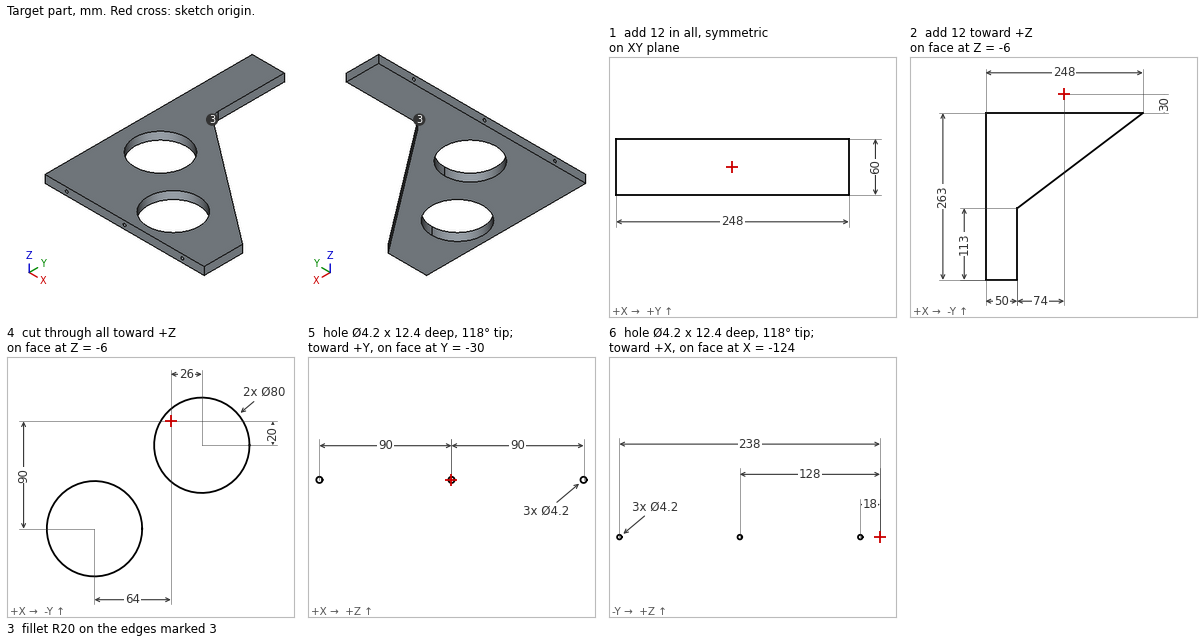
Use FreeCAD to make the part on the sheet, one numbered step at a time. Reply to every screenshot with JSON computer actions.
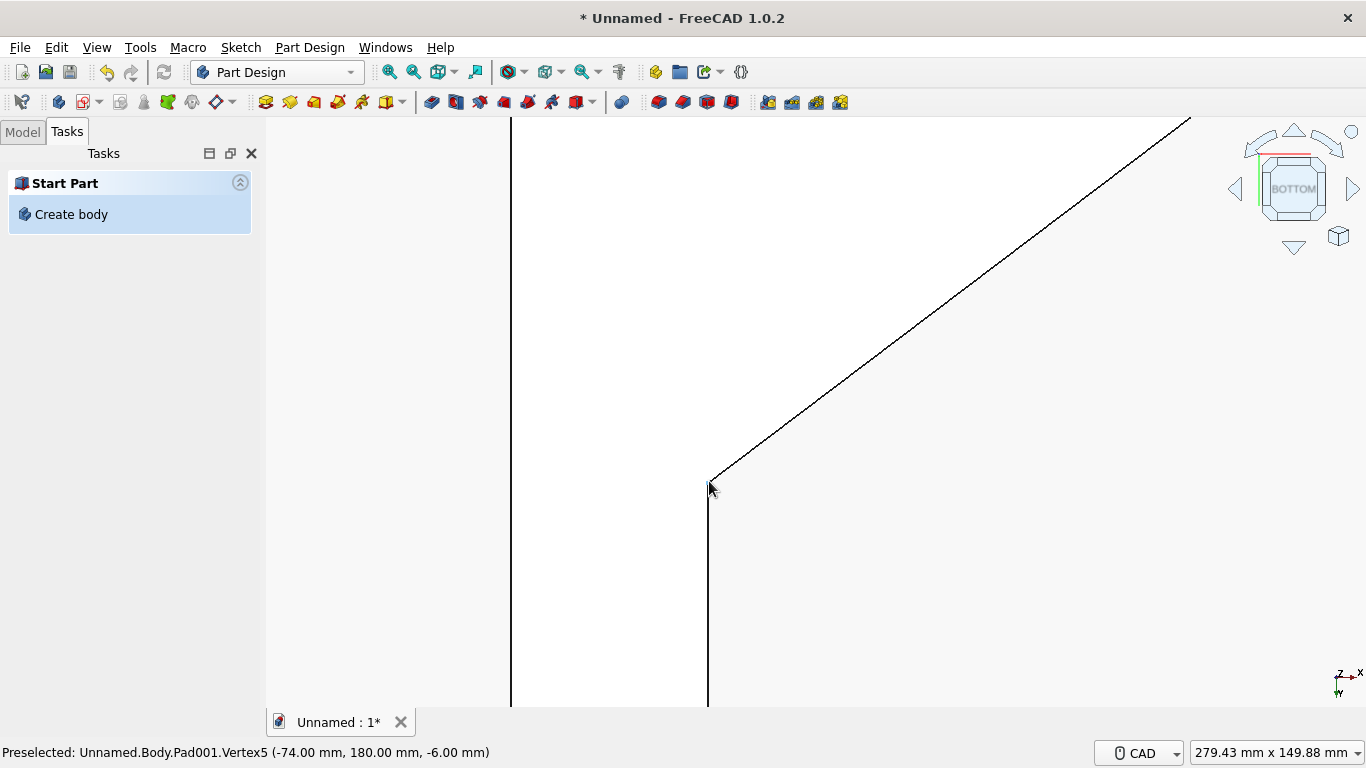
{"action": "key", "text": "v f"}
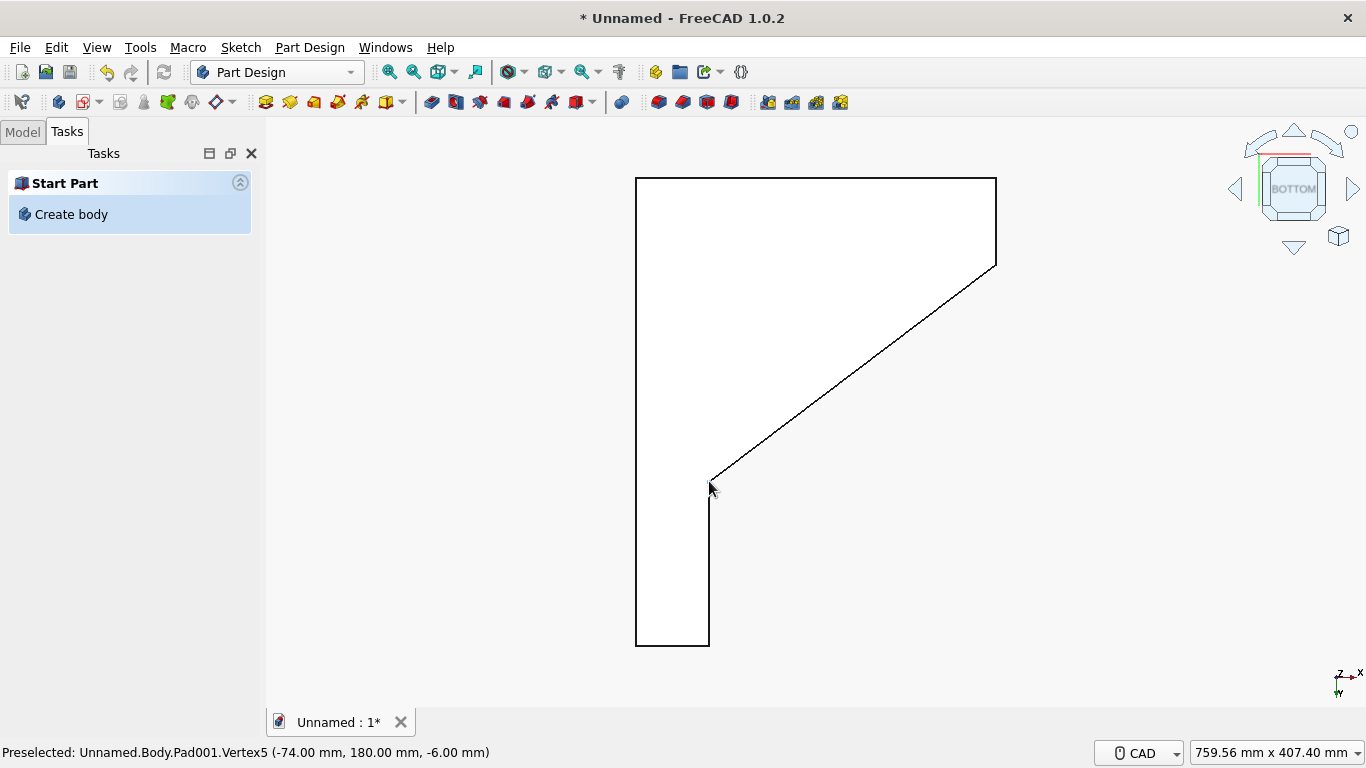
{"action": "key", "text": "0"}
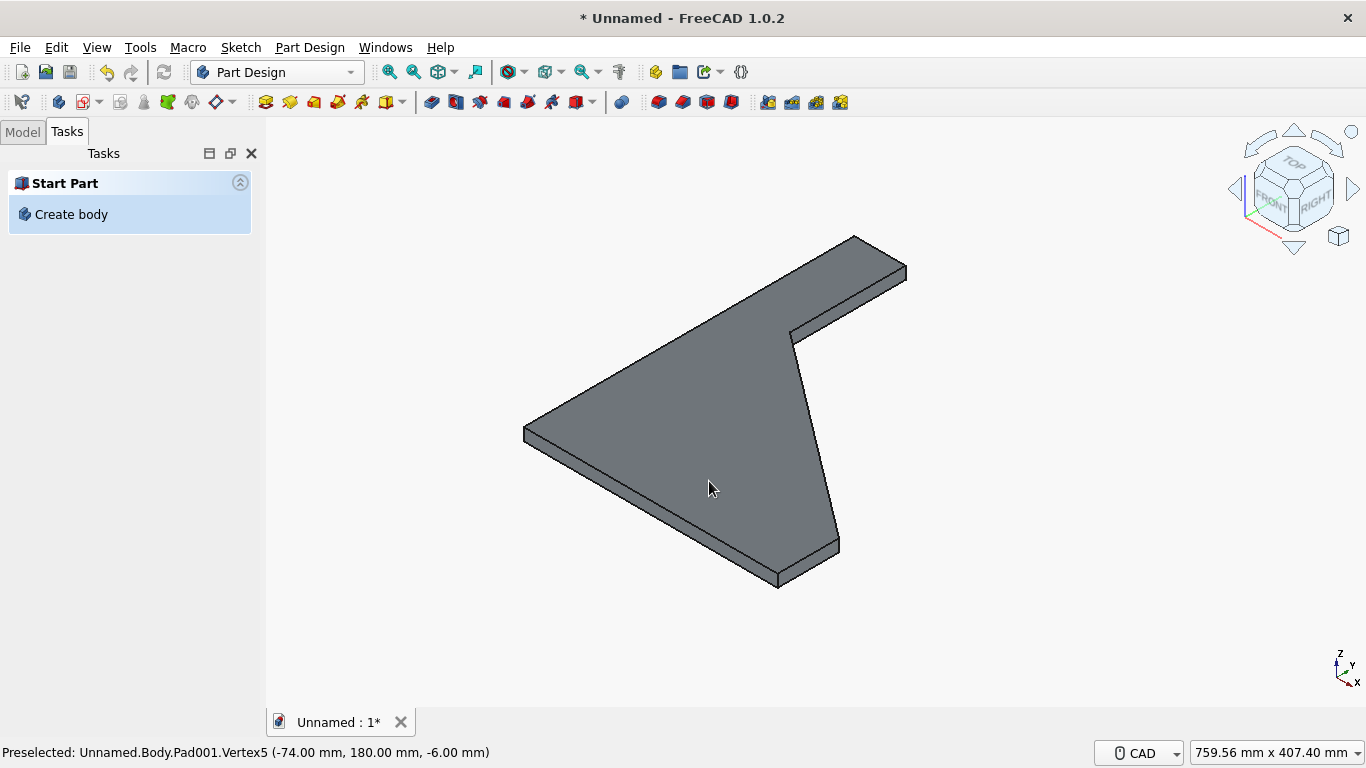
{"action": "scroll", "coordinate": [790, 339], "scroll_direction": "up", "scroll_amount": 5}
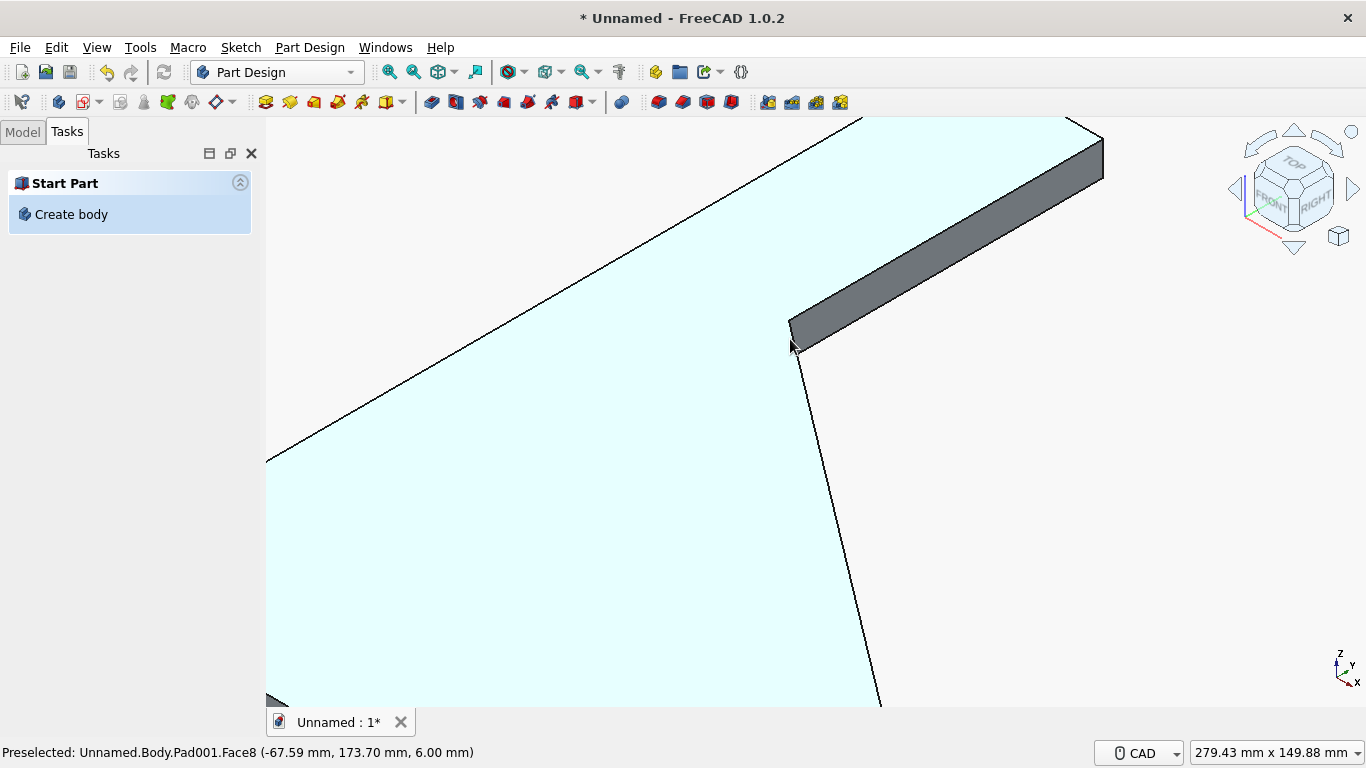
{"action": "key", "text": "v f"}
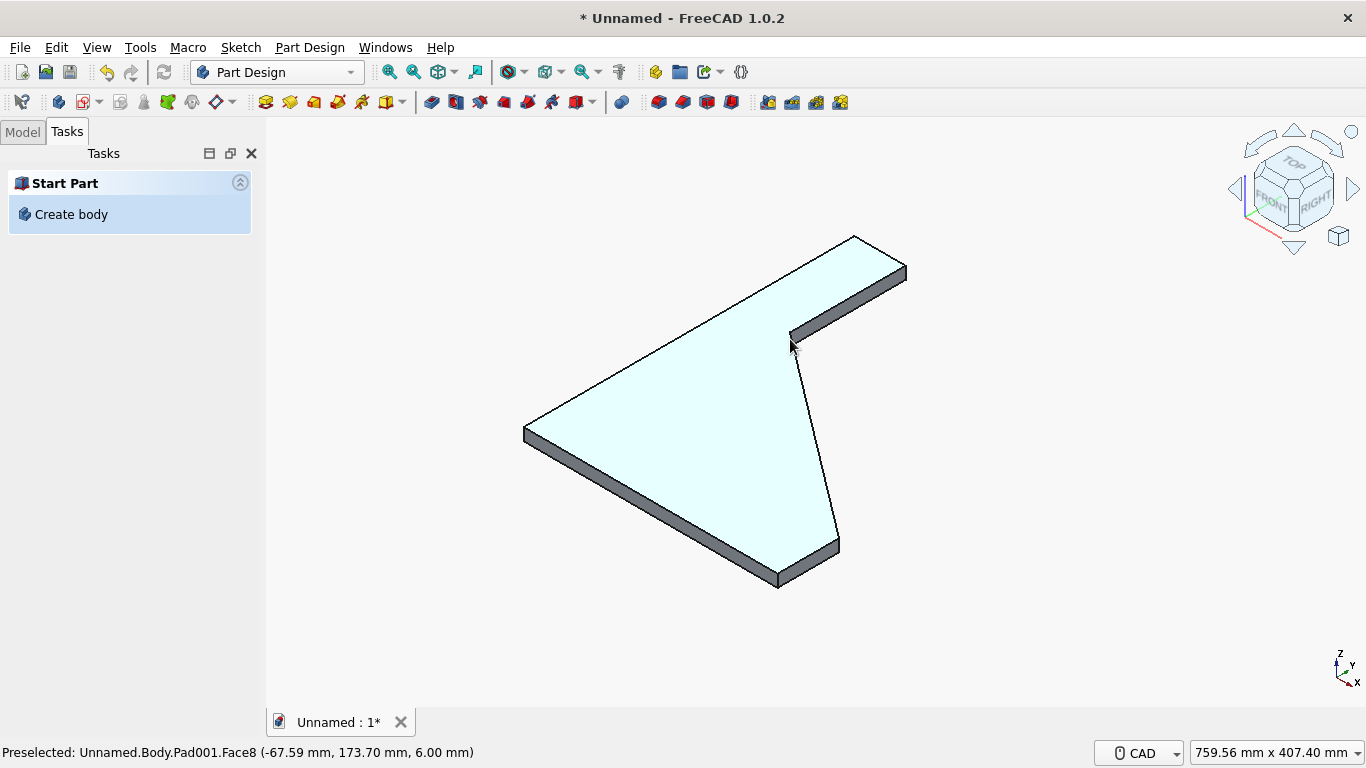
{"action": "key", "text": "2"}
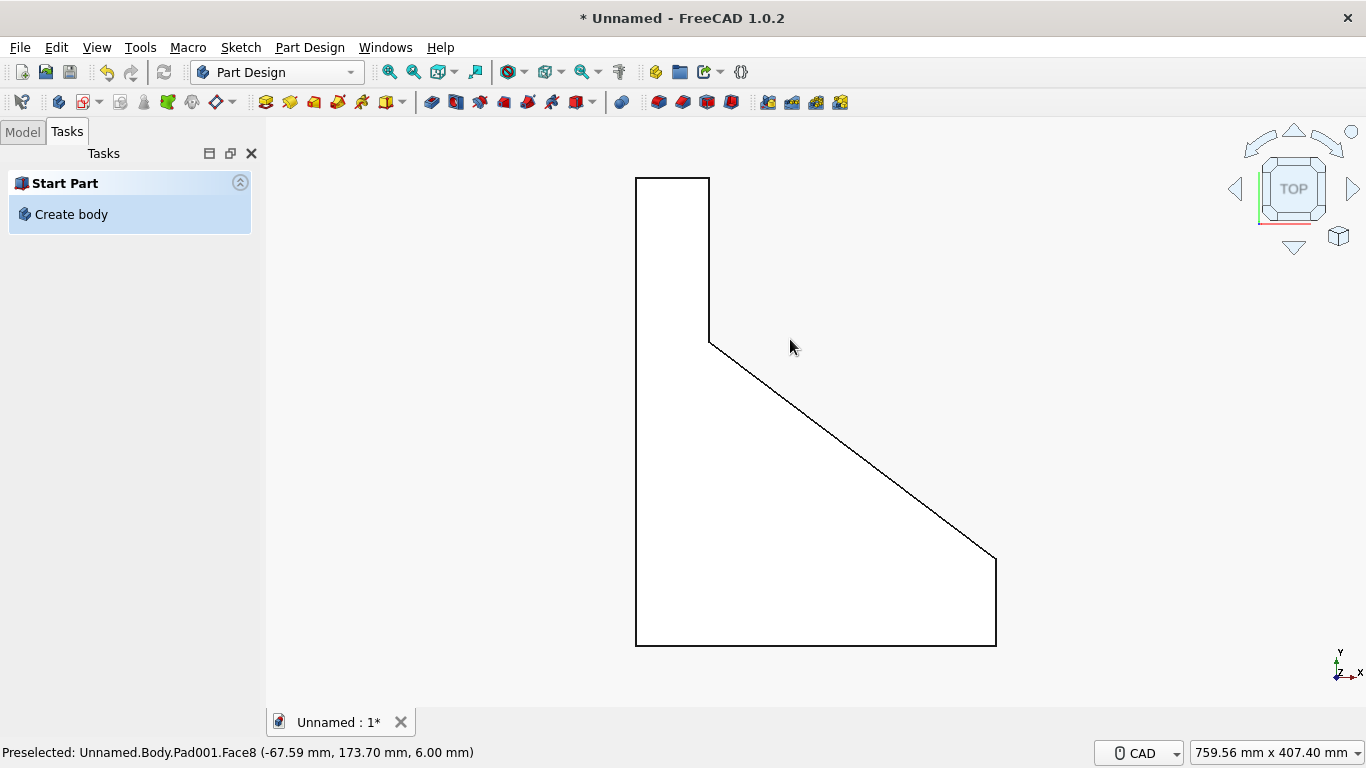
{"action": "scroll", "coordinate": [709, 341], "scroll_direction": "up", "scroll_amount": 5}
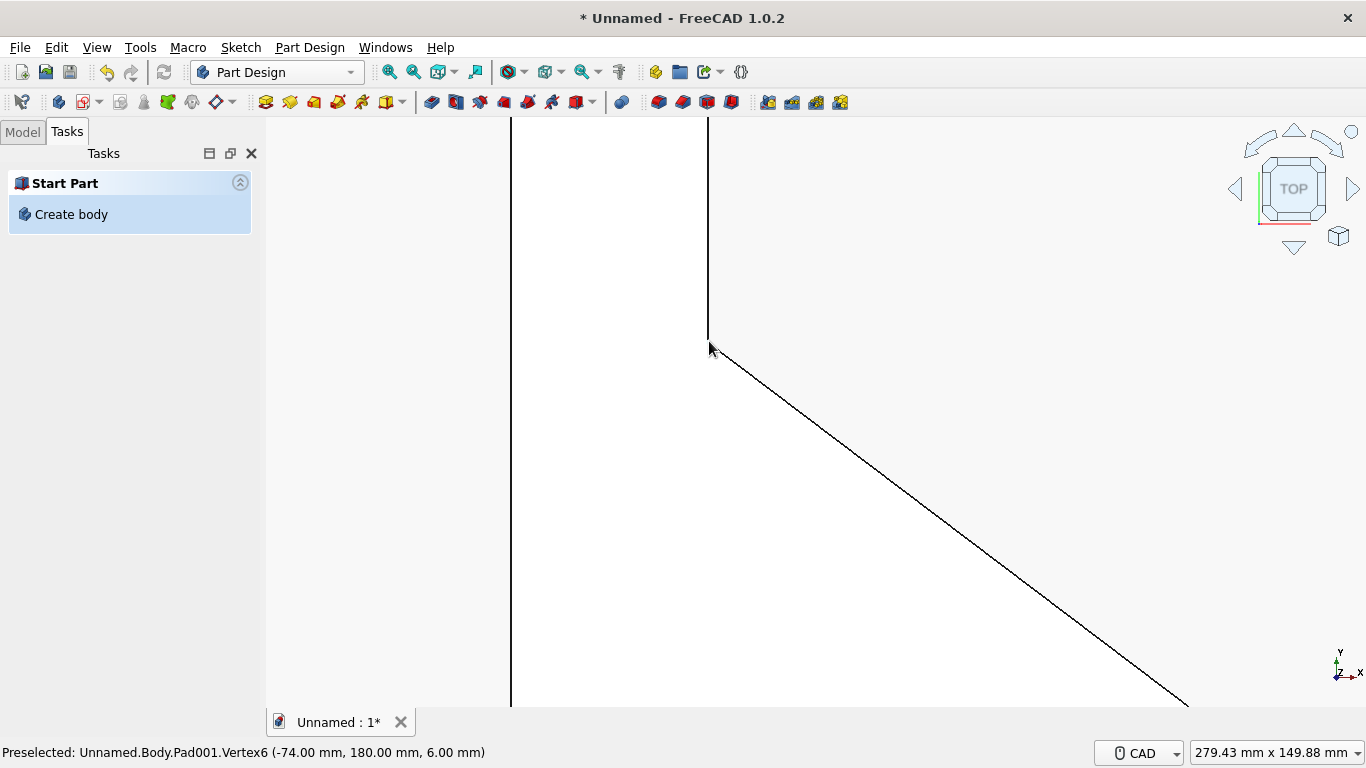
{"action": "left_click", "coordinate": [390, 72]}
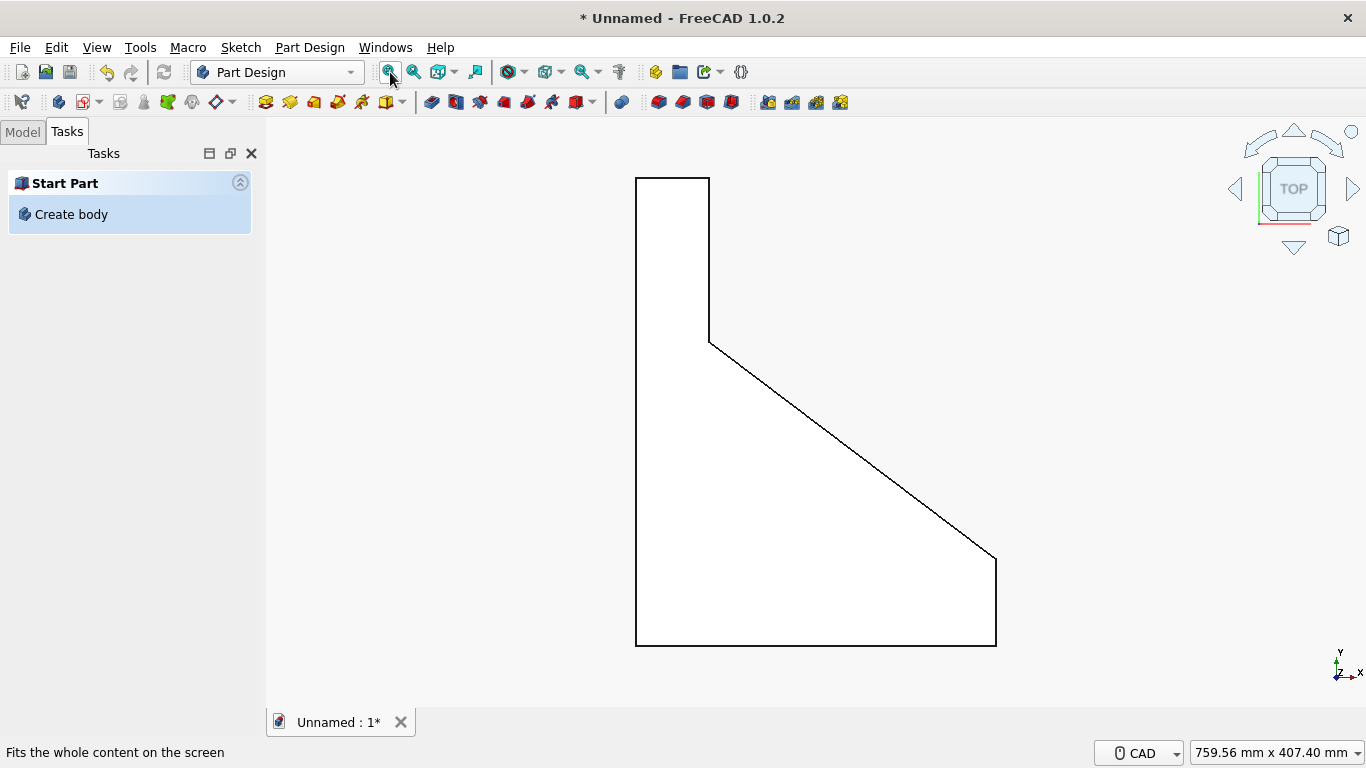
{"action": "key", "text": "1"}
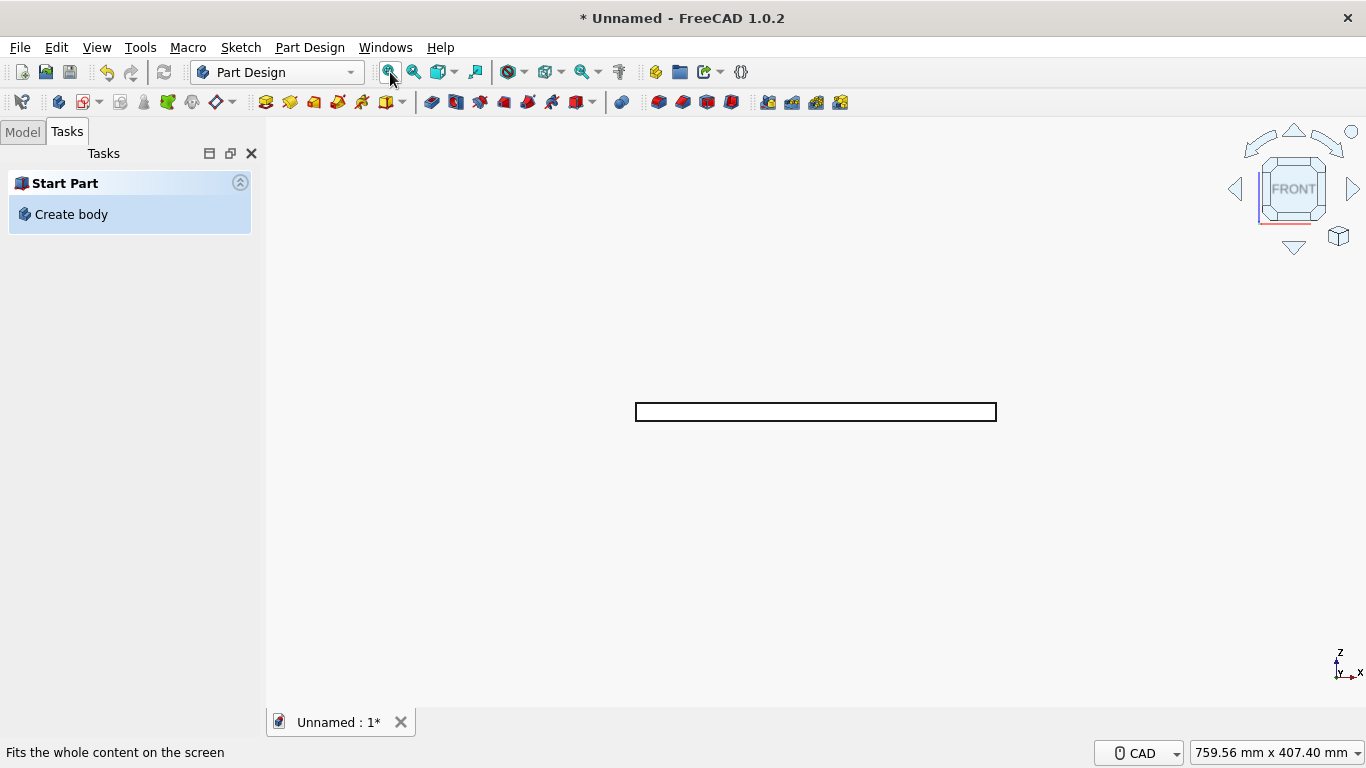
{"action": "key", "text": "v f"}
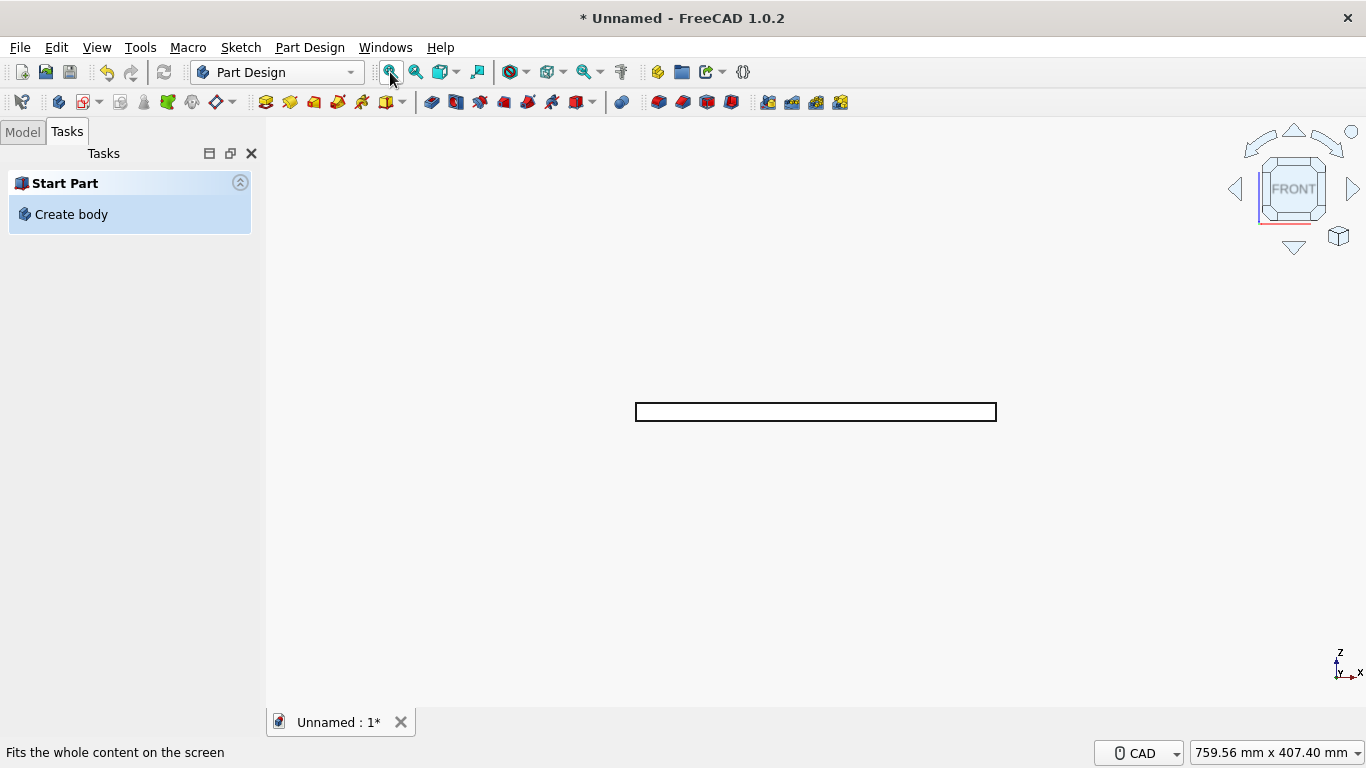
{"action": "scroll", "coordinate": [709, 411], "scroll_direction": "up", "scroll_amount": 5}